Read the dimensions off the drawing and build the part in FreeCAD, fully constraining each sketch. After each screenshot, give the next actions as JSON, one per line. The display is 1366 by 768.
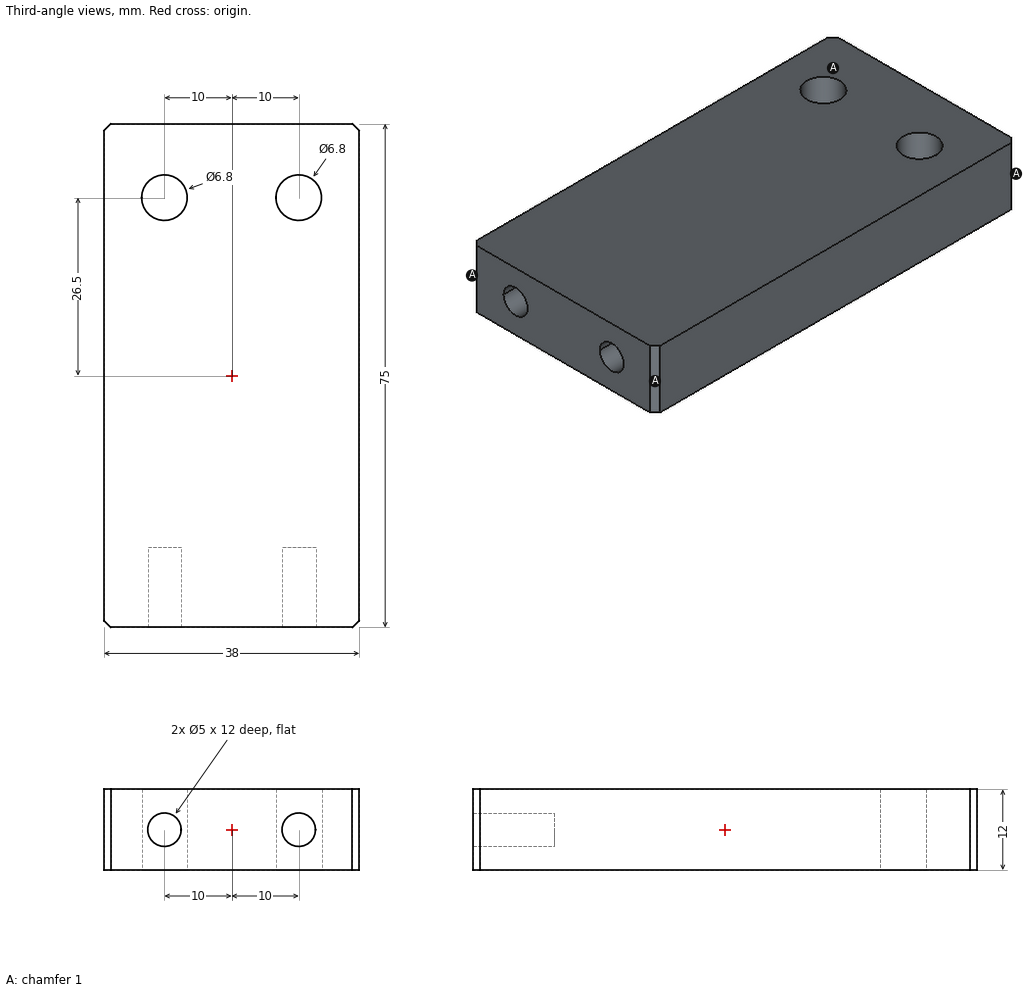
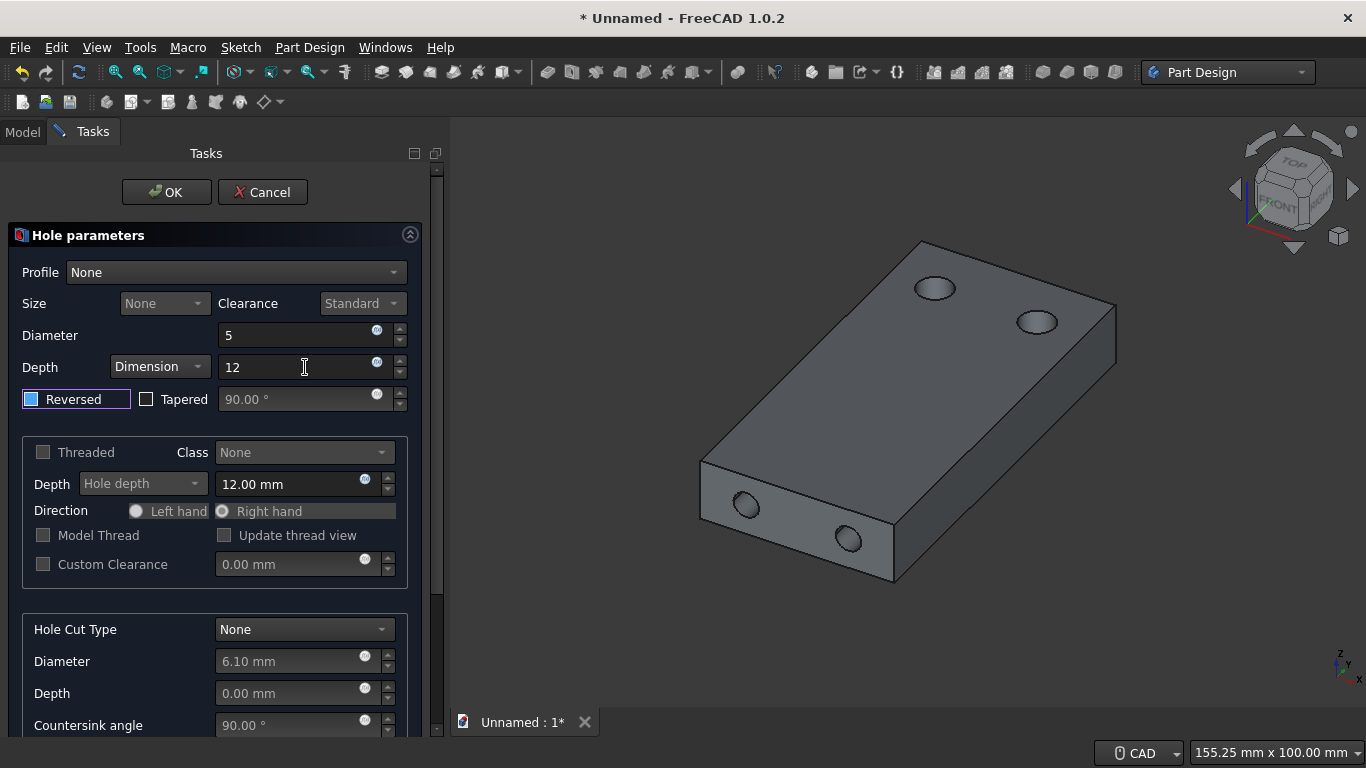
{"action": "scroll", "coordinate": [437, 450], "scroll_direction": "down", "scroll_amount": 3}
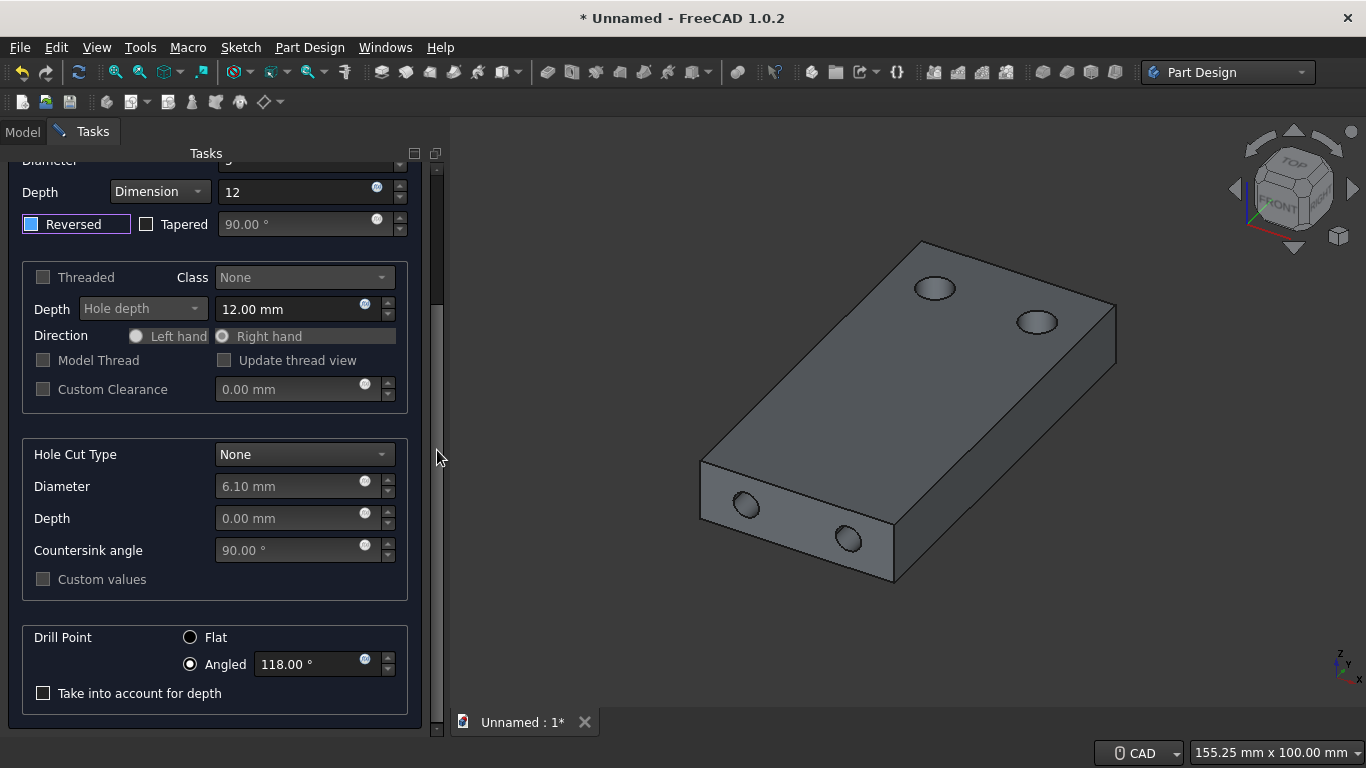
{"action": "left_click", "coordinate": [191, 637]}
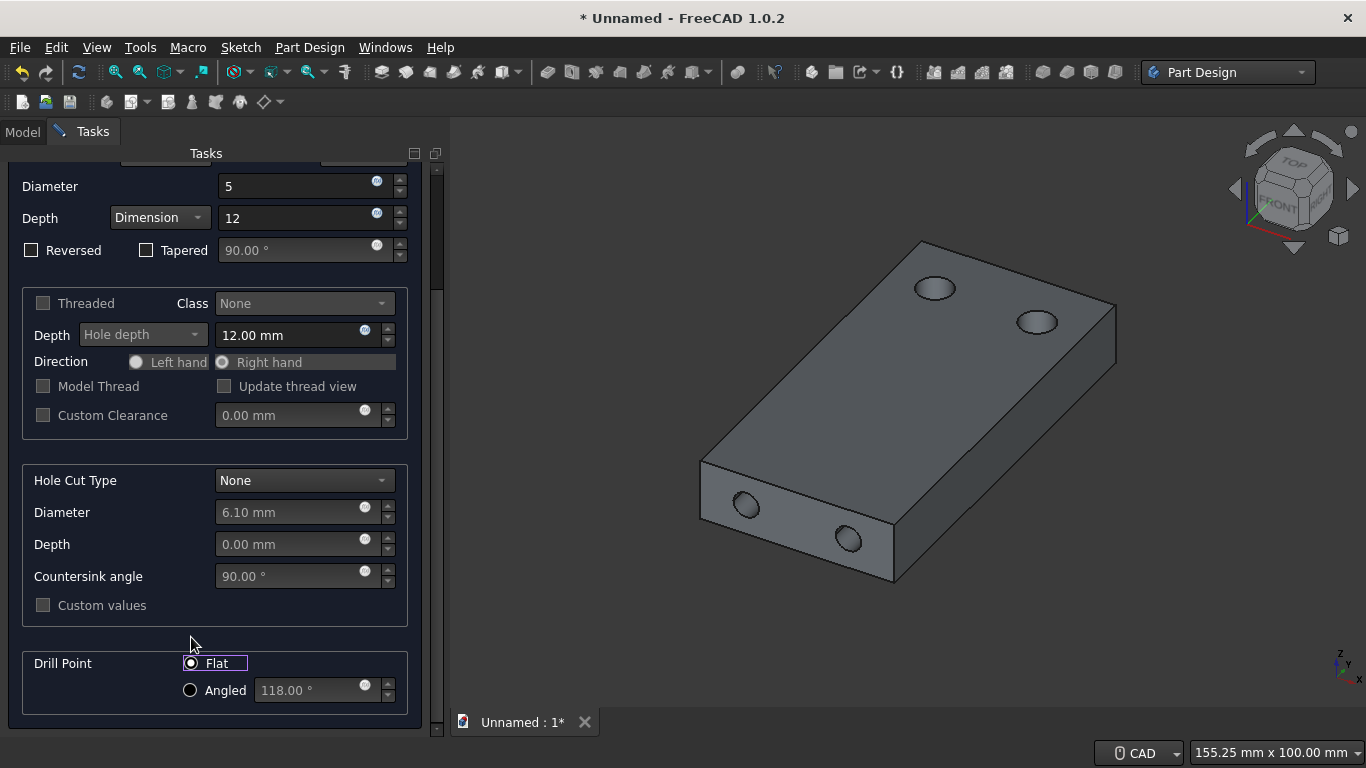
{"action": "scroll", "coordinate": [437, 450], "scroll_direction": "up", "scroll_amount": 4}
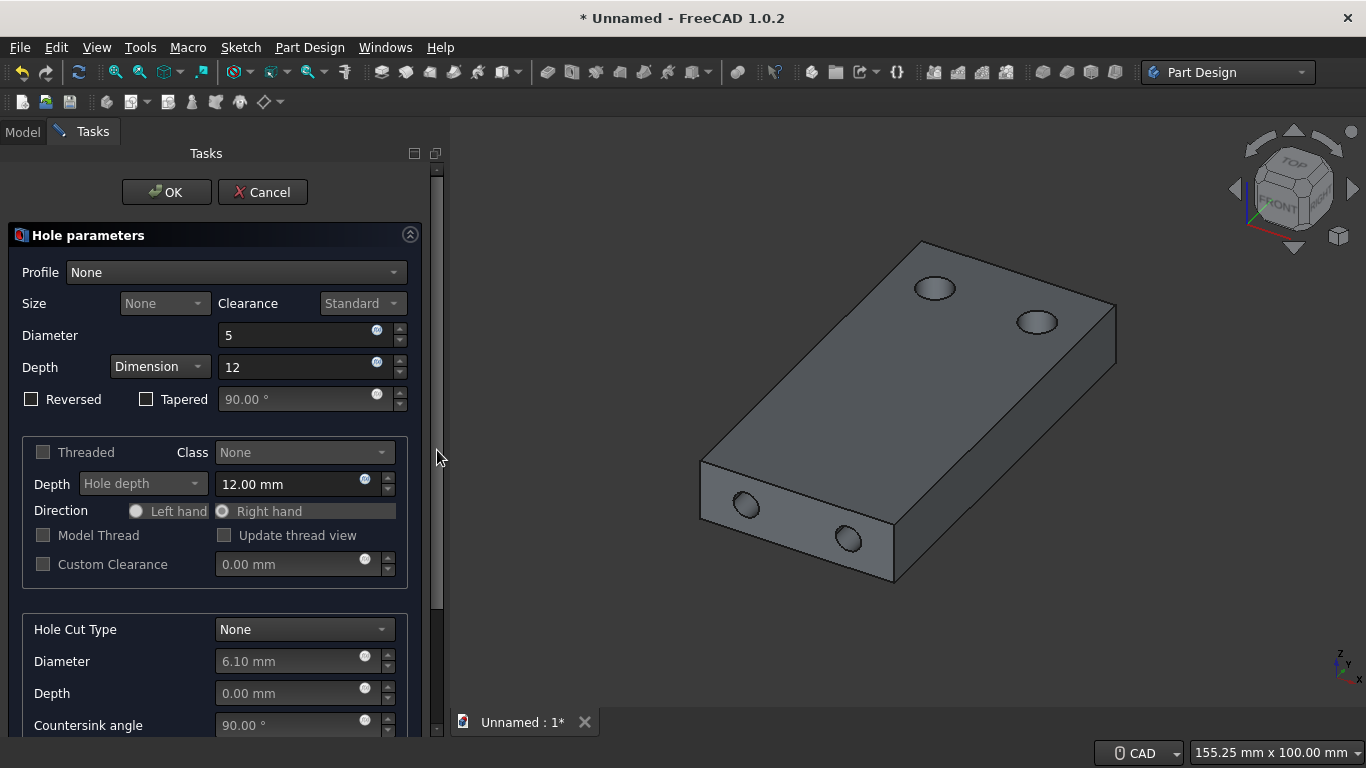
{"action": "left_click", "coordinate": [167, 192]}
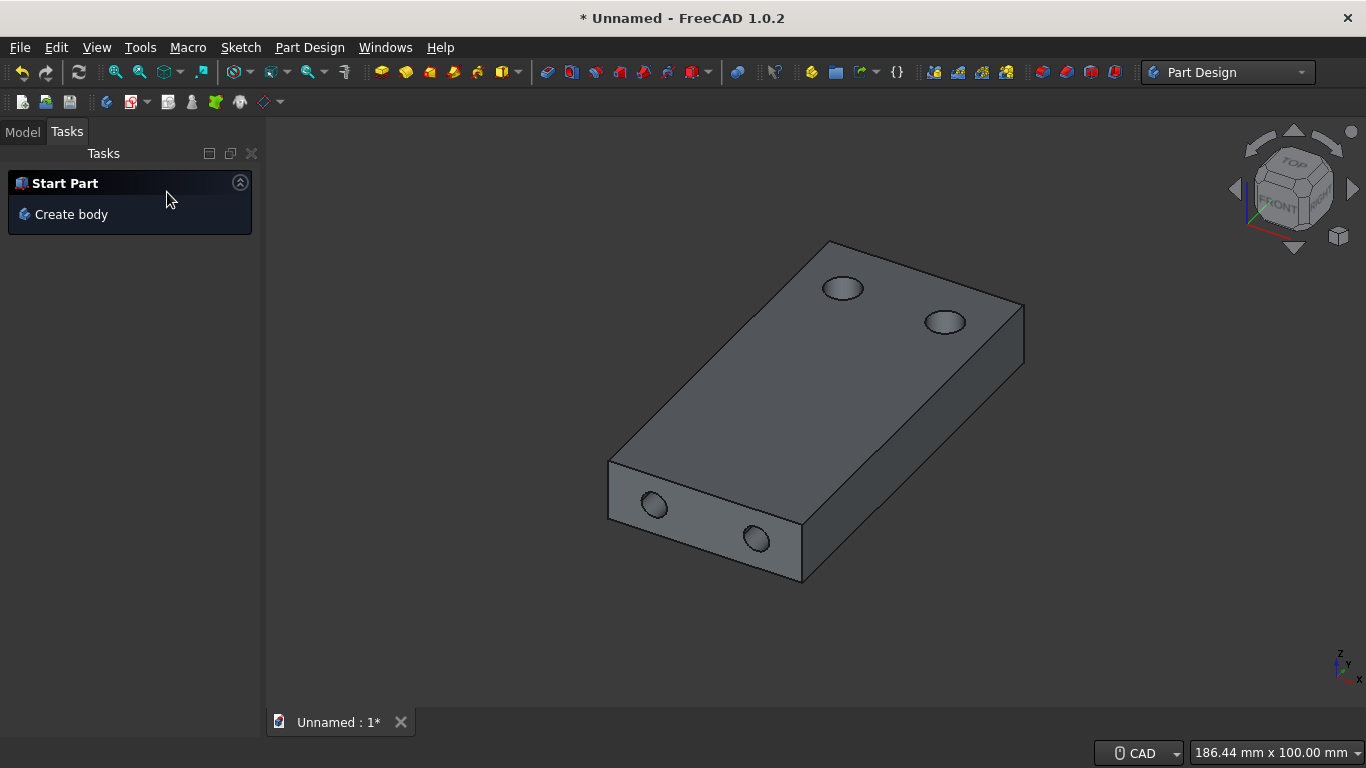
{"action": "left_click", "coordinate": [802, 553]}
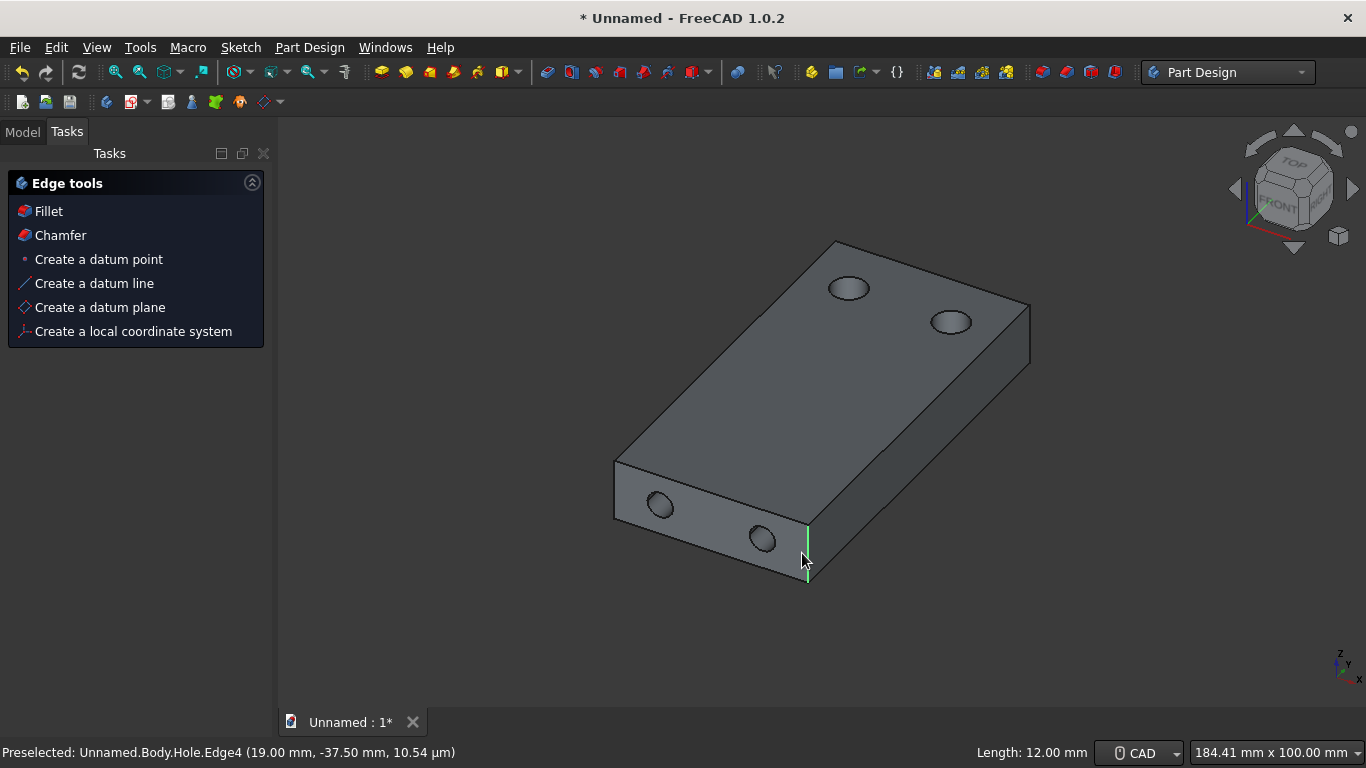
{"action": "key", "text": "0"}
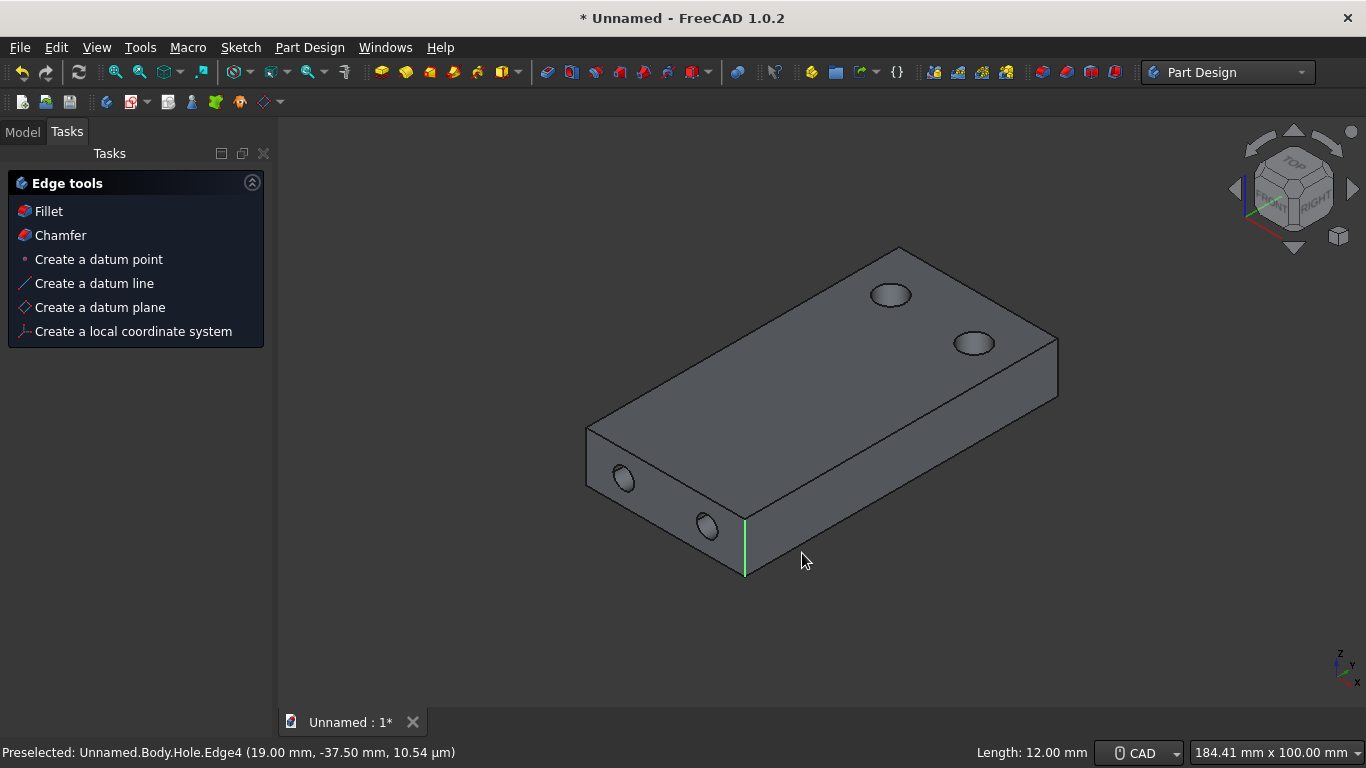
{"action": "key", "text": "2"}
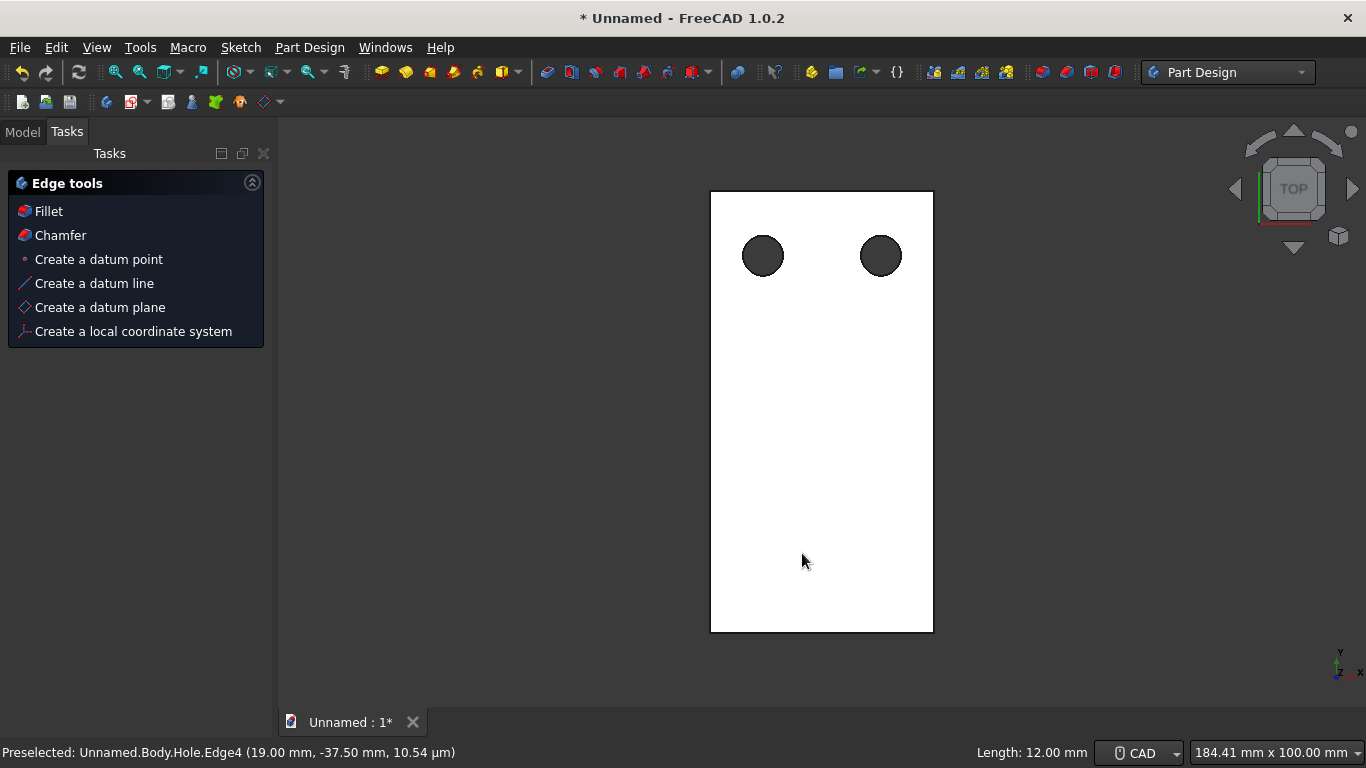
{"action": "key", "text": "1"}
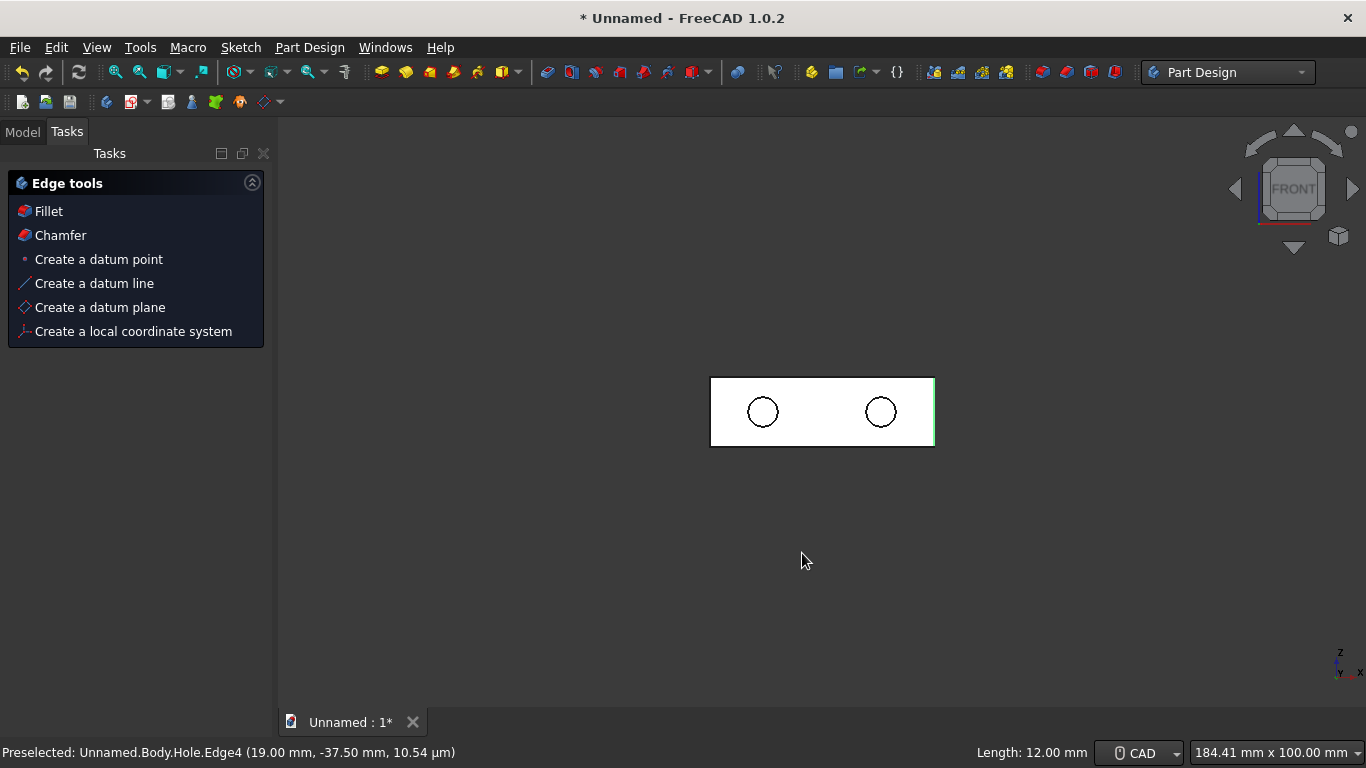
{"action": "left_click", "coordinate": [116, 72]}